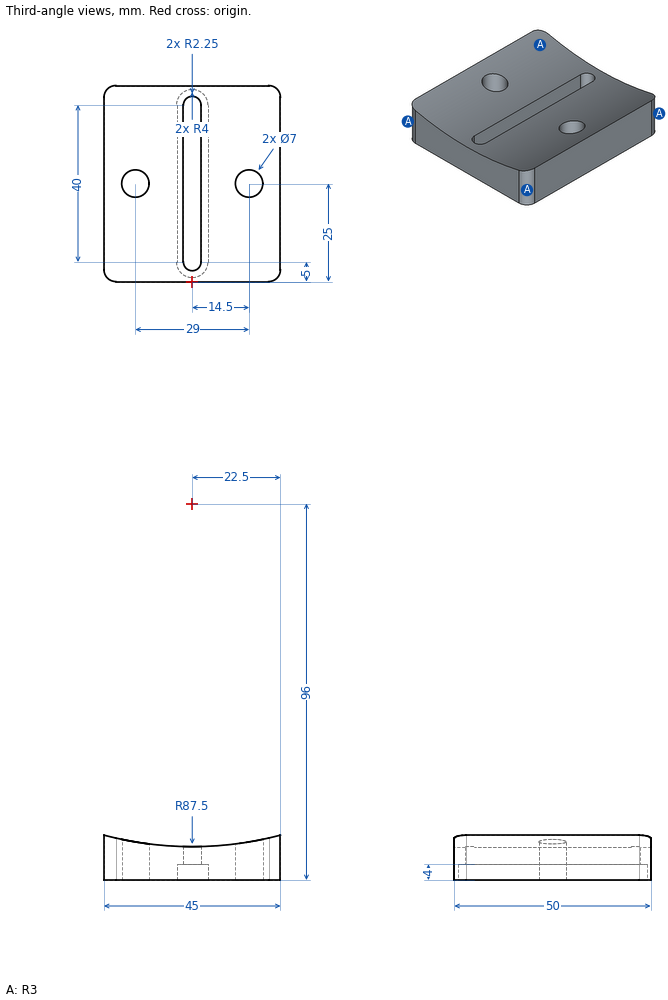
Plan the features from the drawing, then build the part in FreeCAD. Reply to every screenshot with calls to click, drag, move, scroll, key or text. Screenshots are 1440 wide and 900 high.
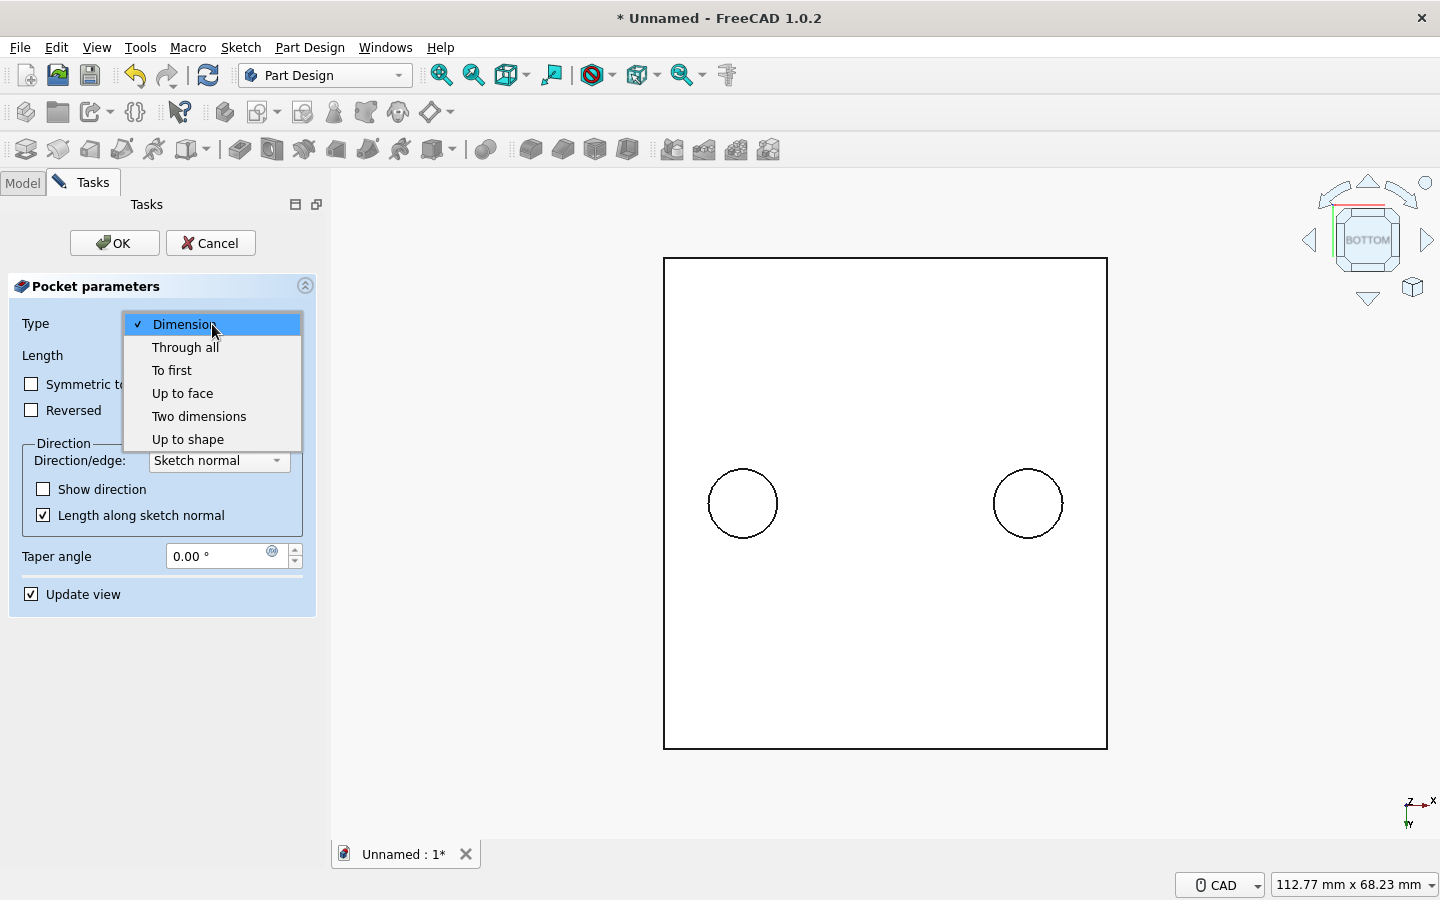
click(212, 348)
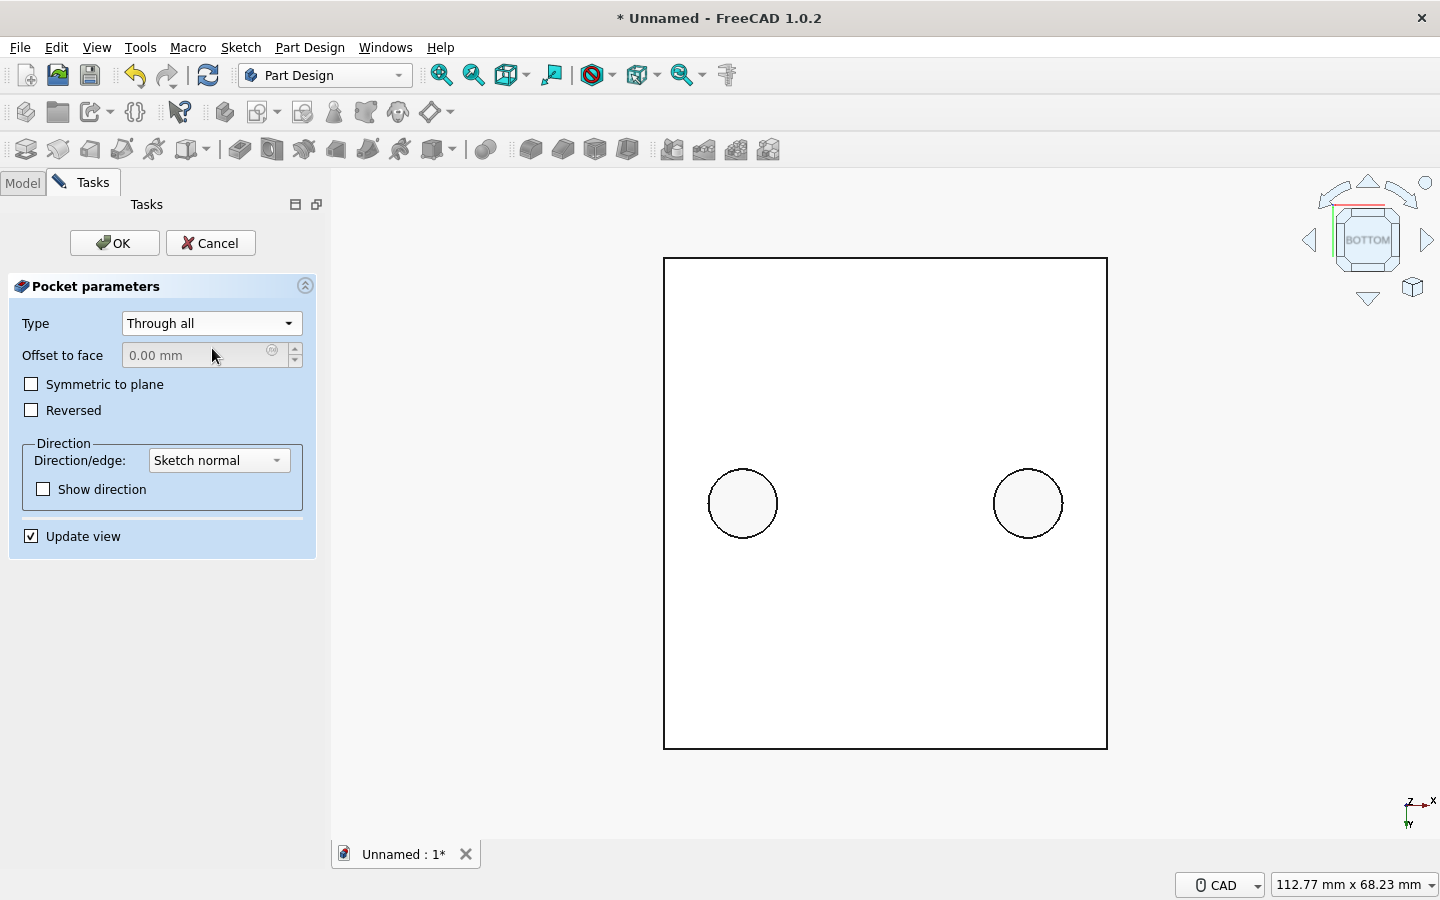
click(115, 243)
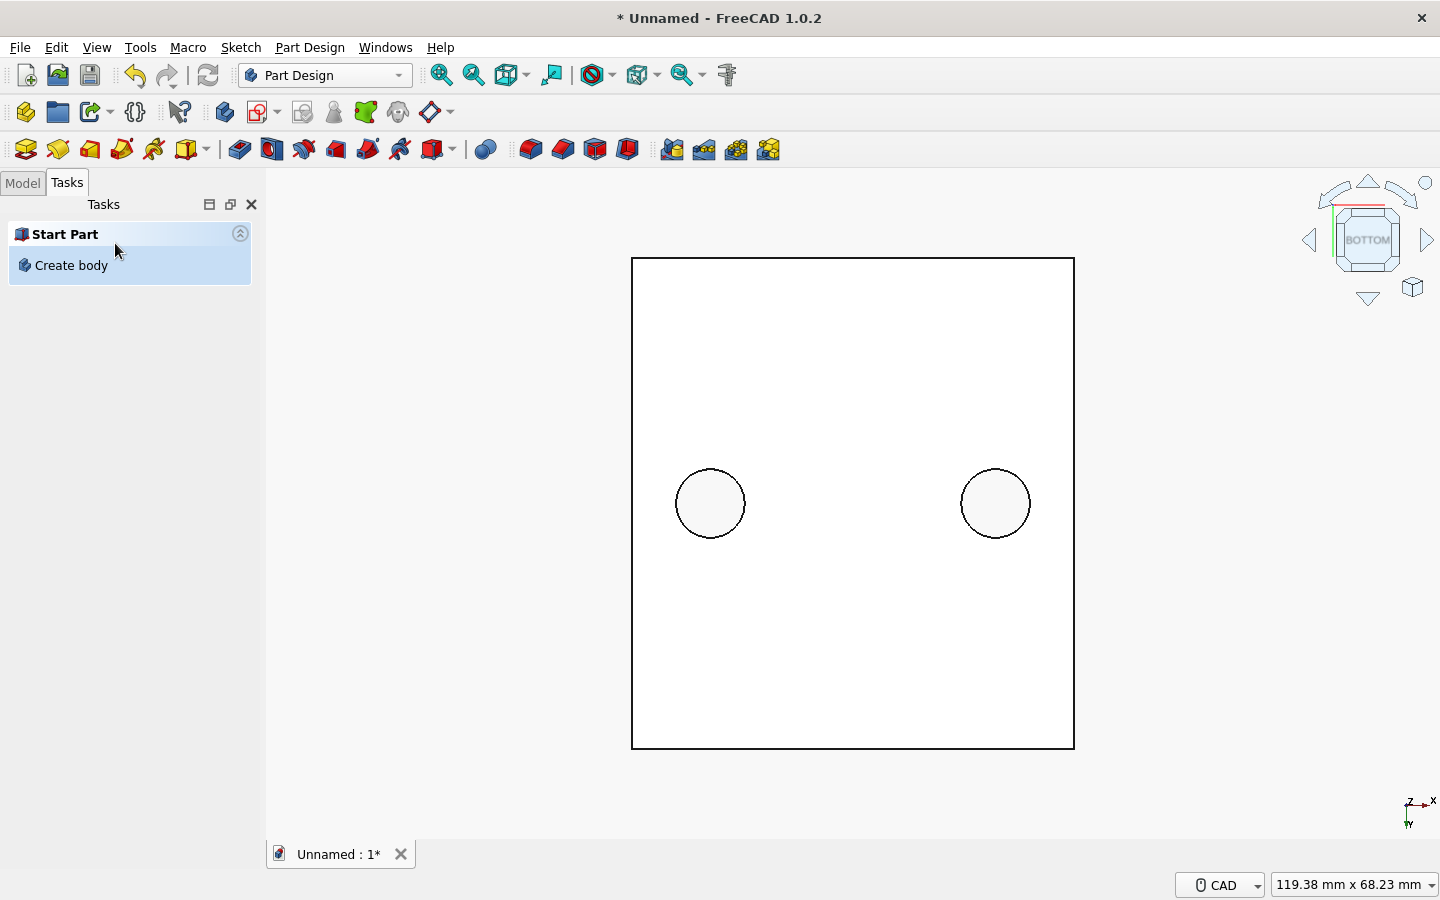
click(853, 432)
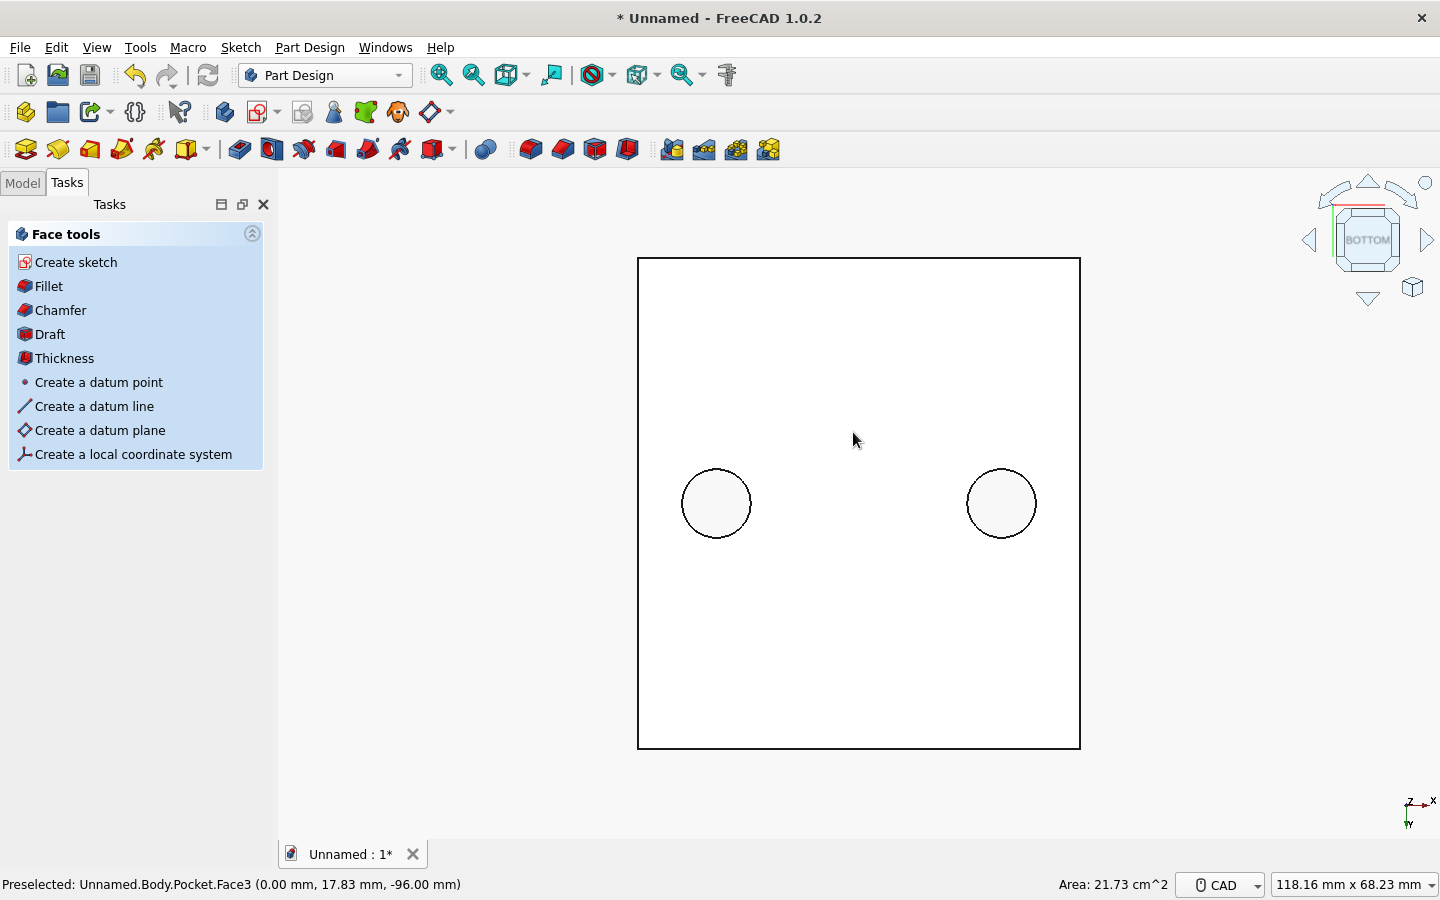
click(258, 112)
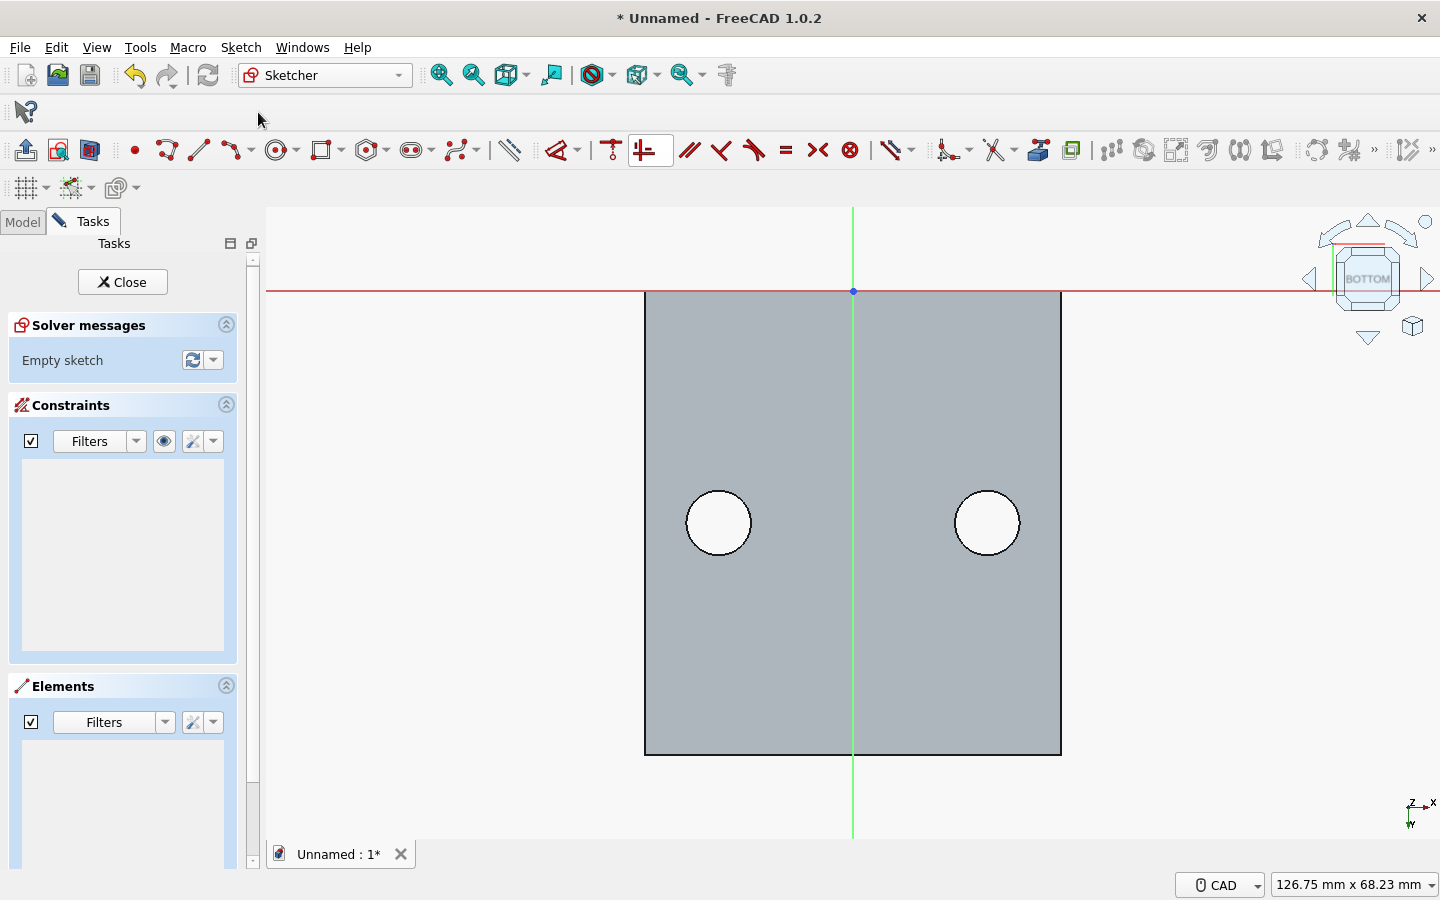
key(g)
key(s)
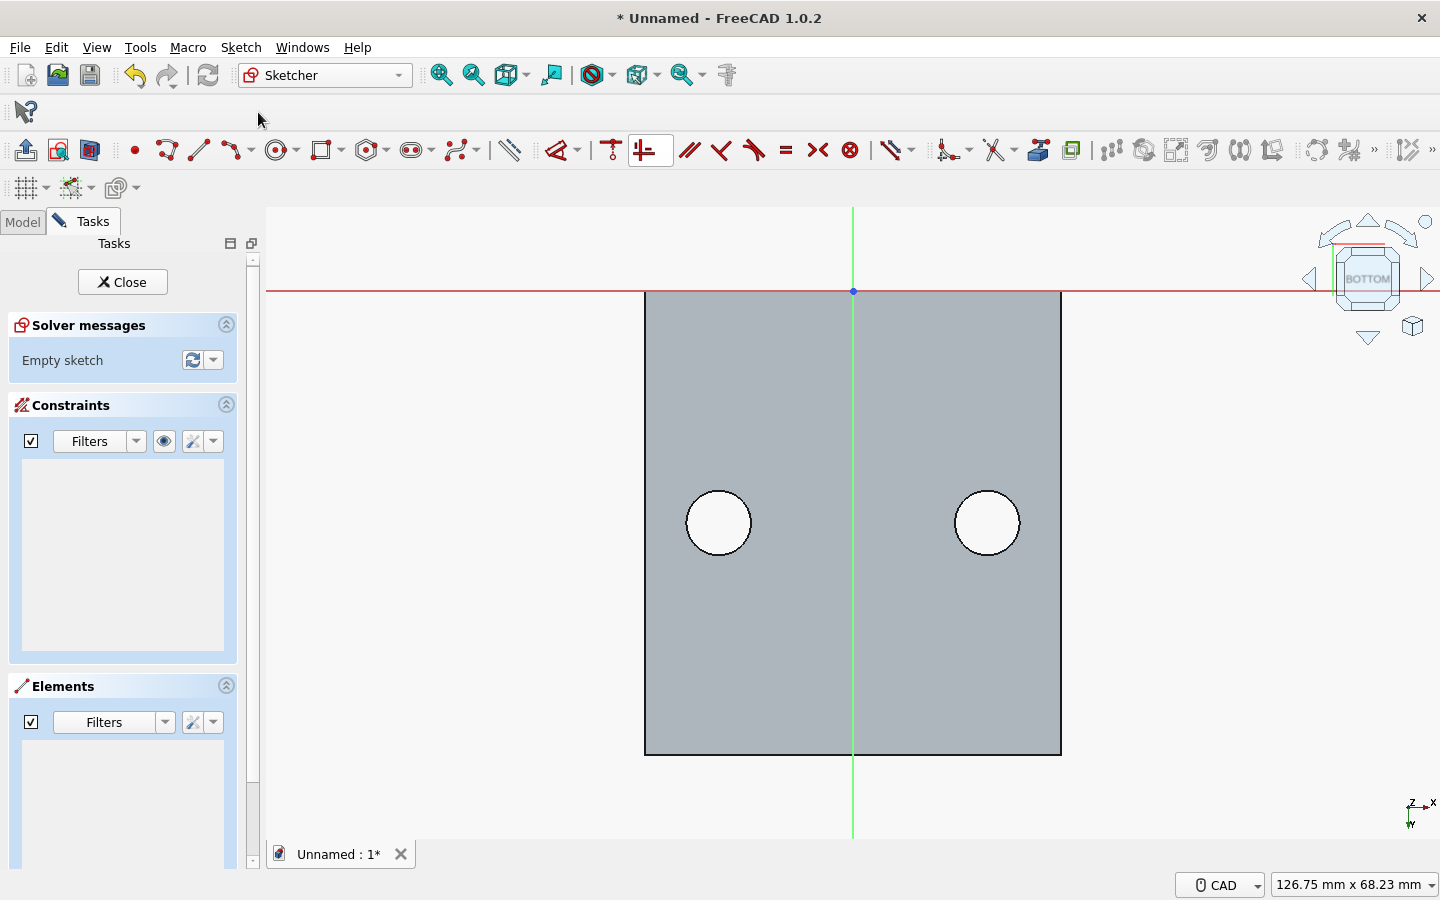
click(853, 708)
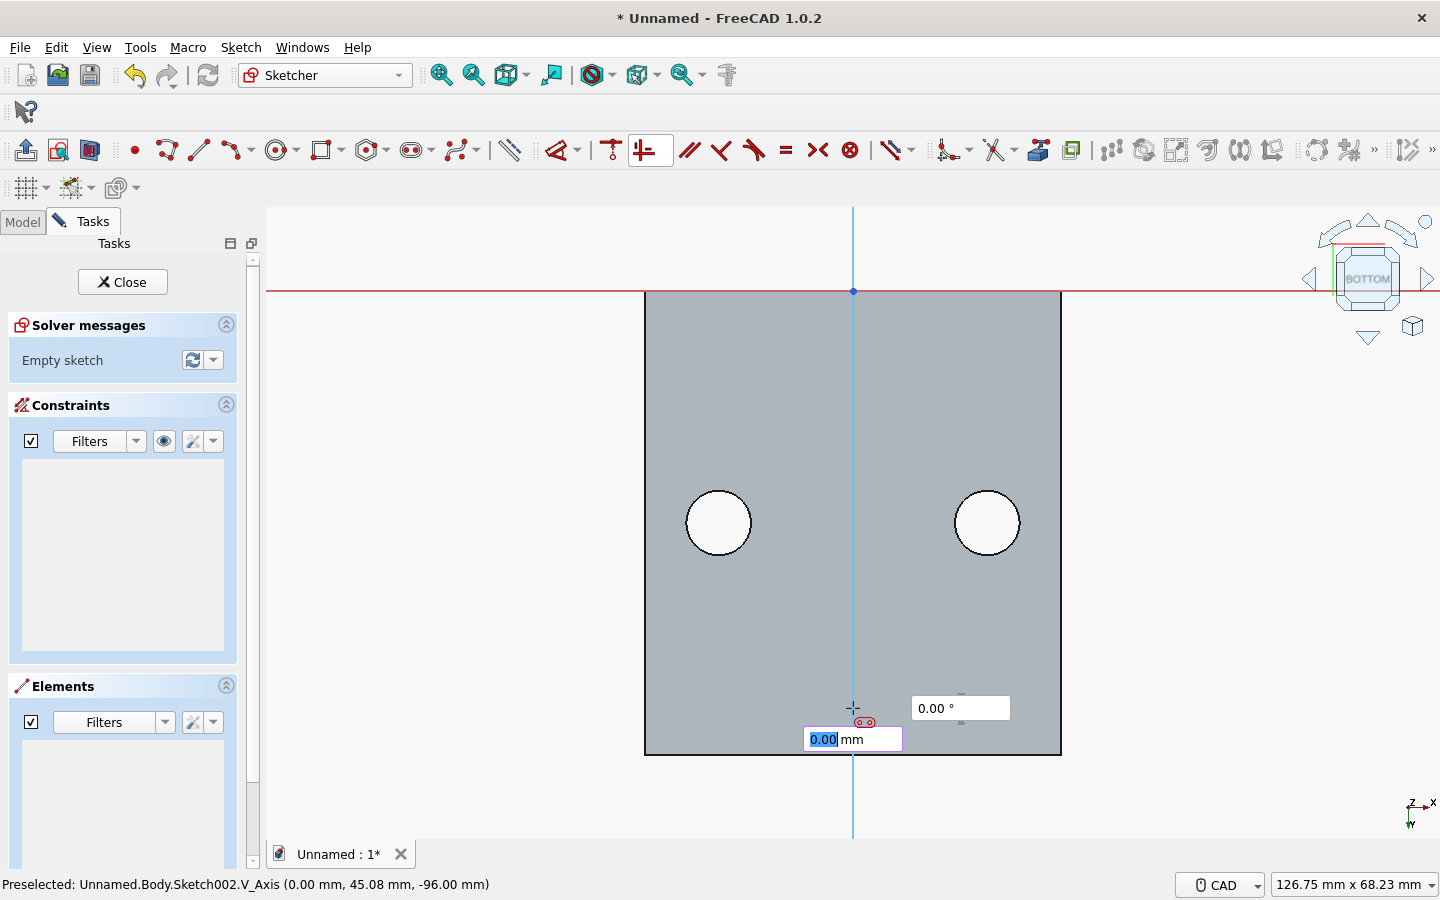
click(862, 338)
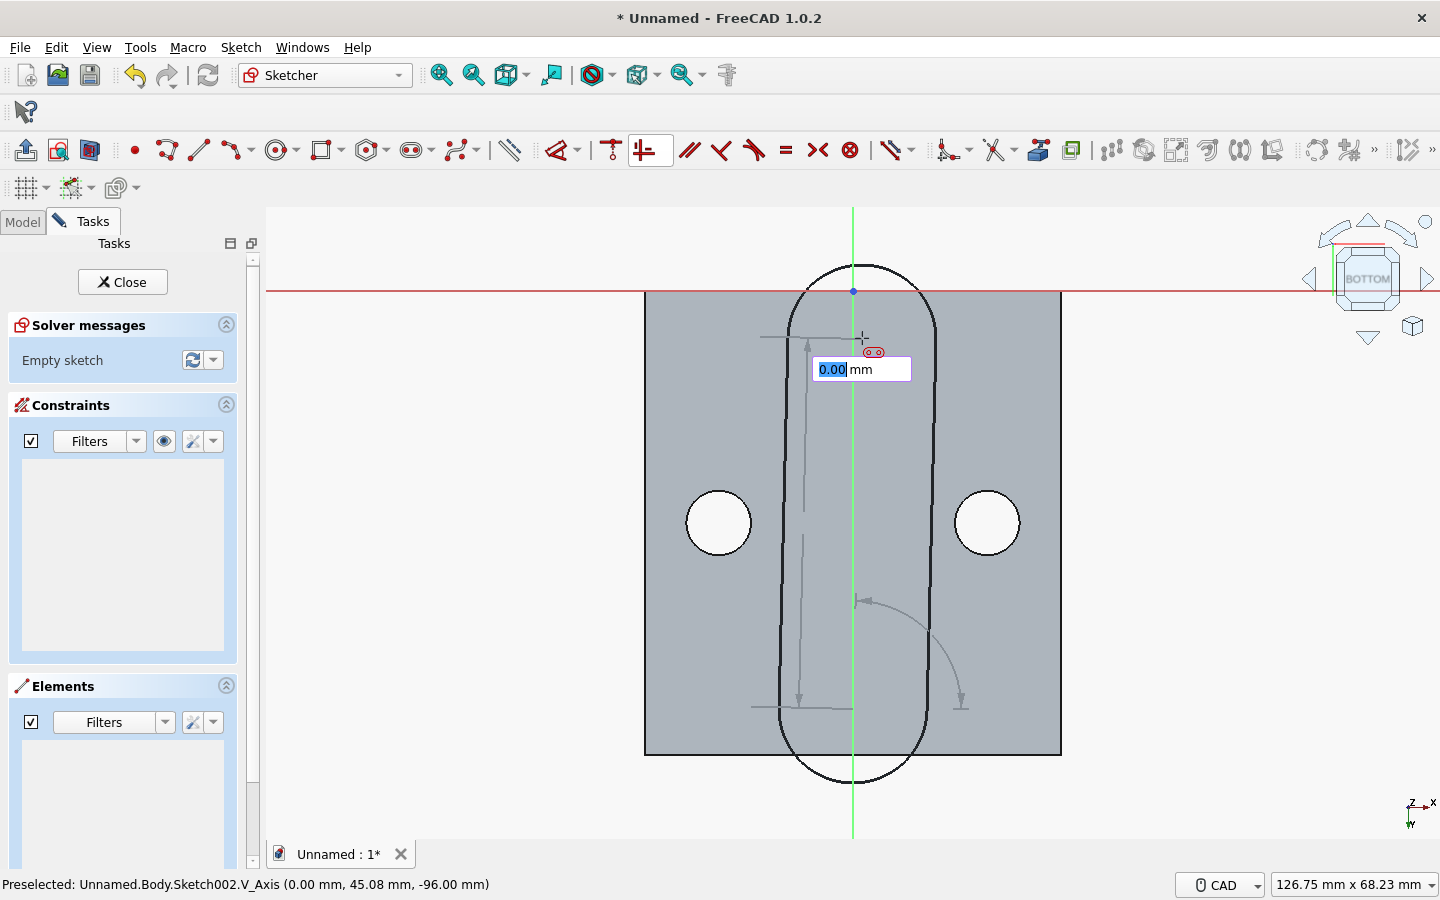
click(832, 523)
key(Escape)